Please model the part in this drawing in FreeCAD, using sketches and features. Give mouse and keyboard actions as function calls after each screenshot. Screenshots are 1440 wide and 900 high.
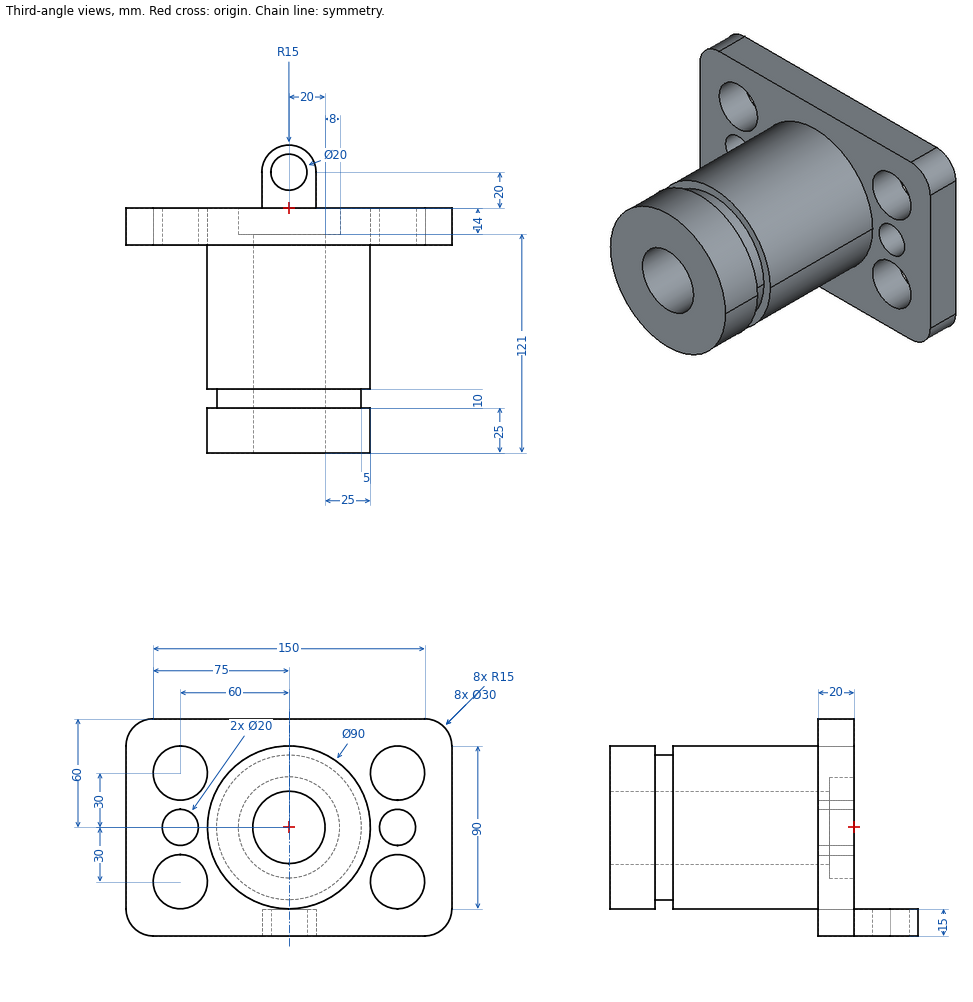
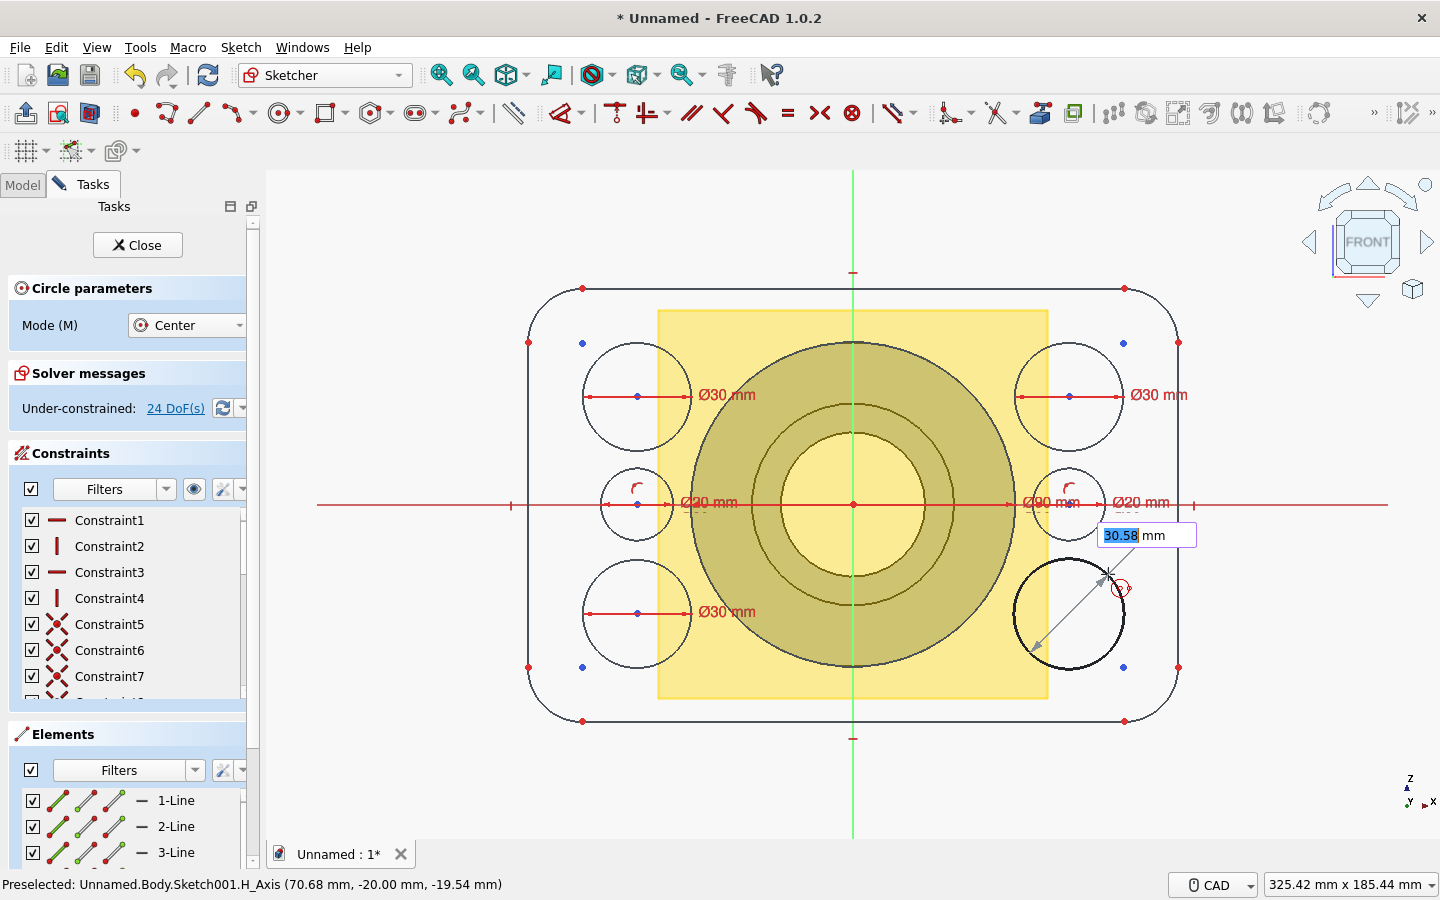
text(30)
key(Return)
key(Escape)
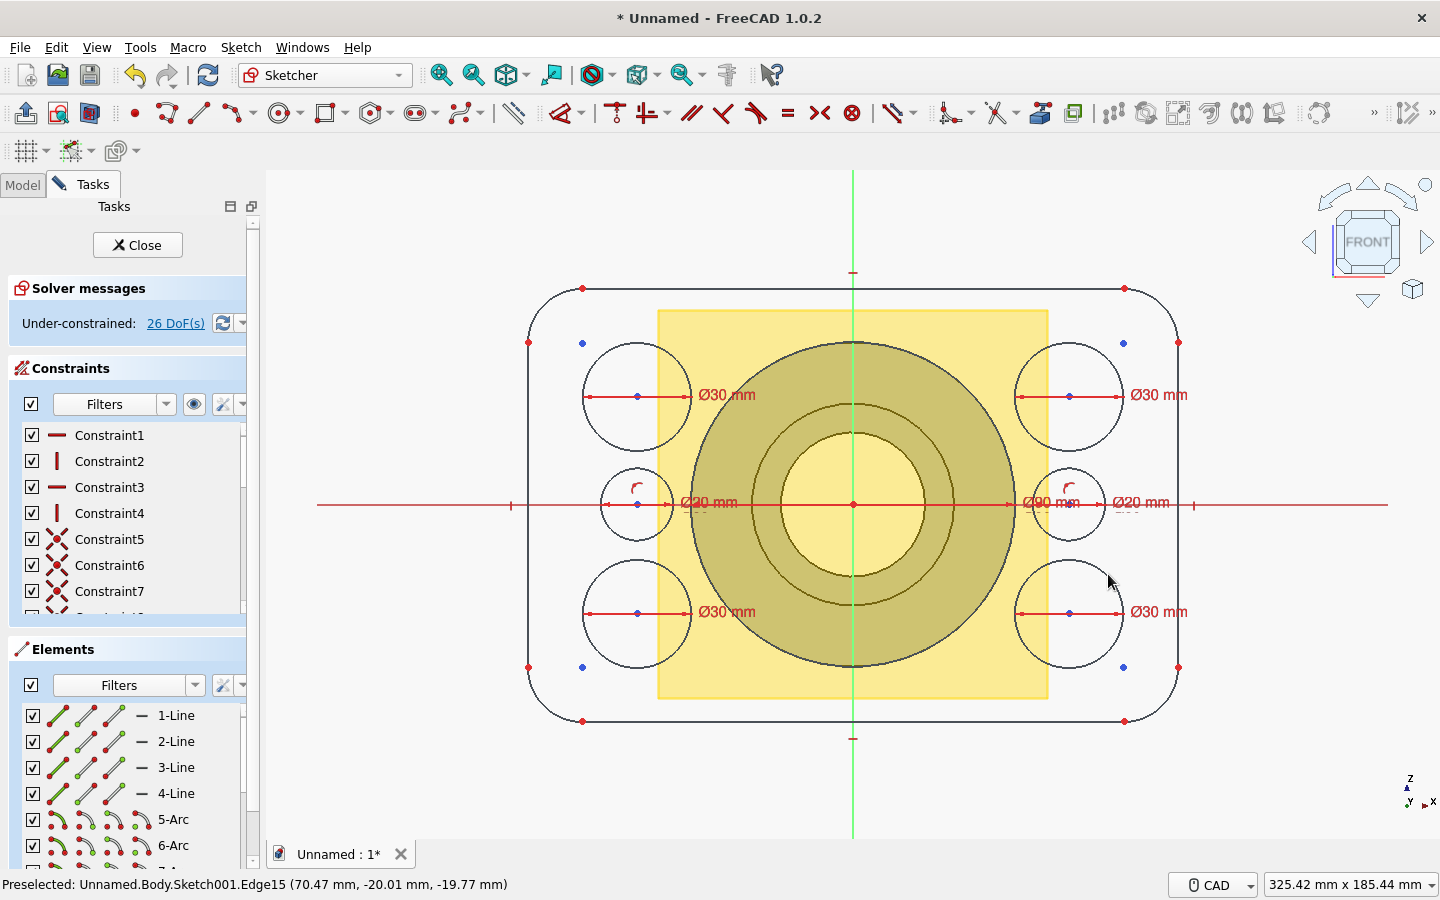
click(745, 289)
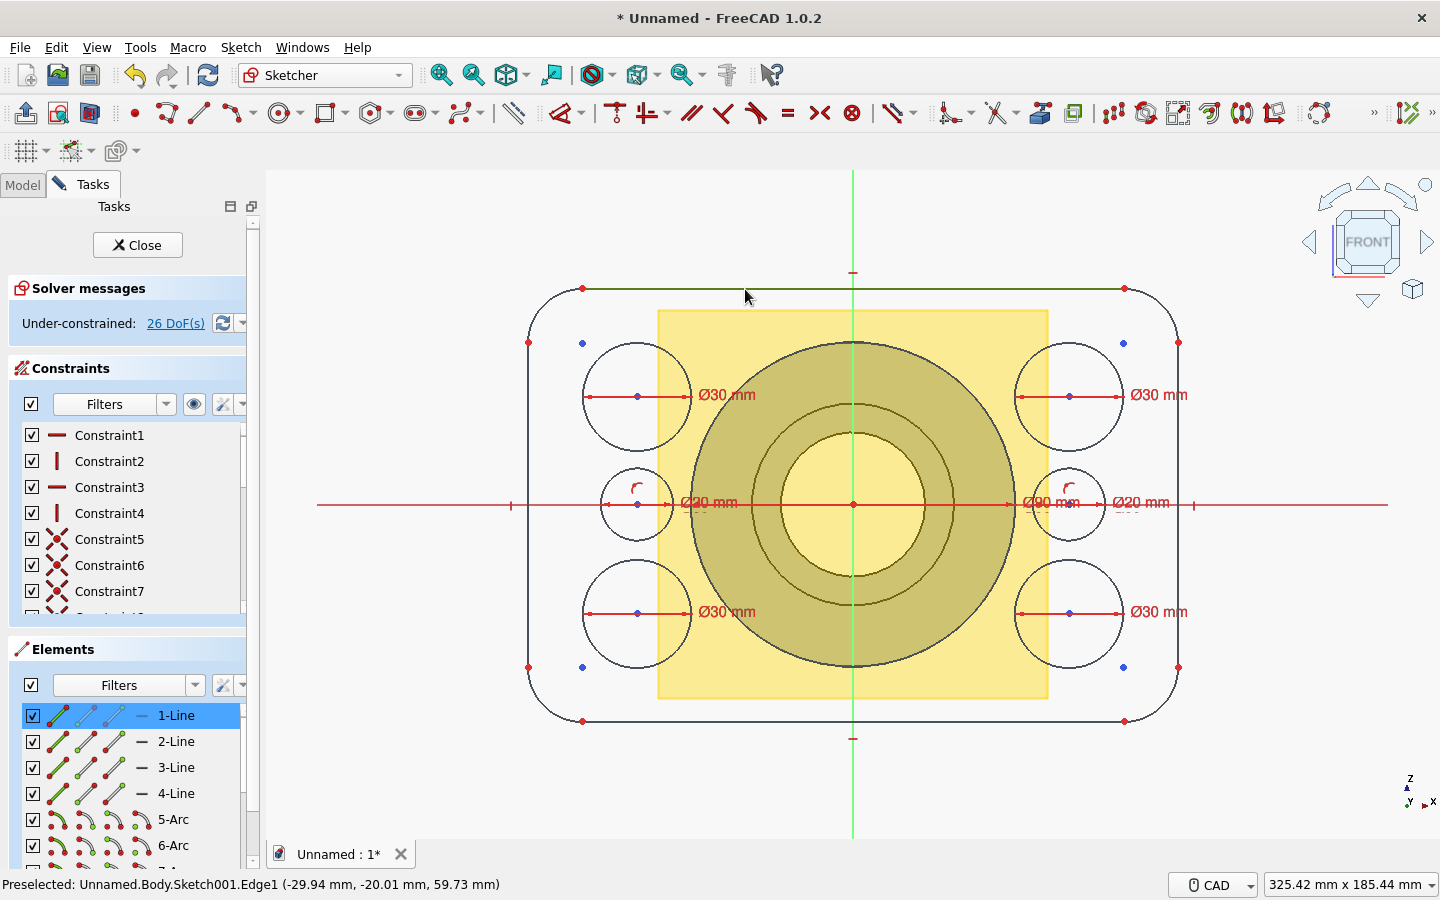
click(1172, 319)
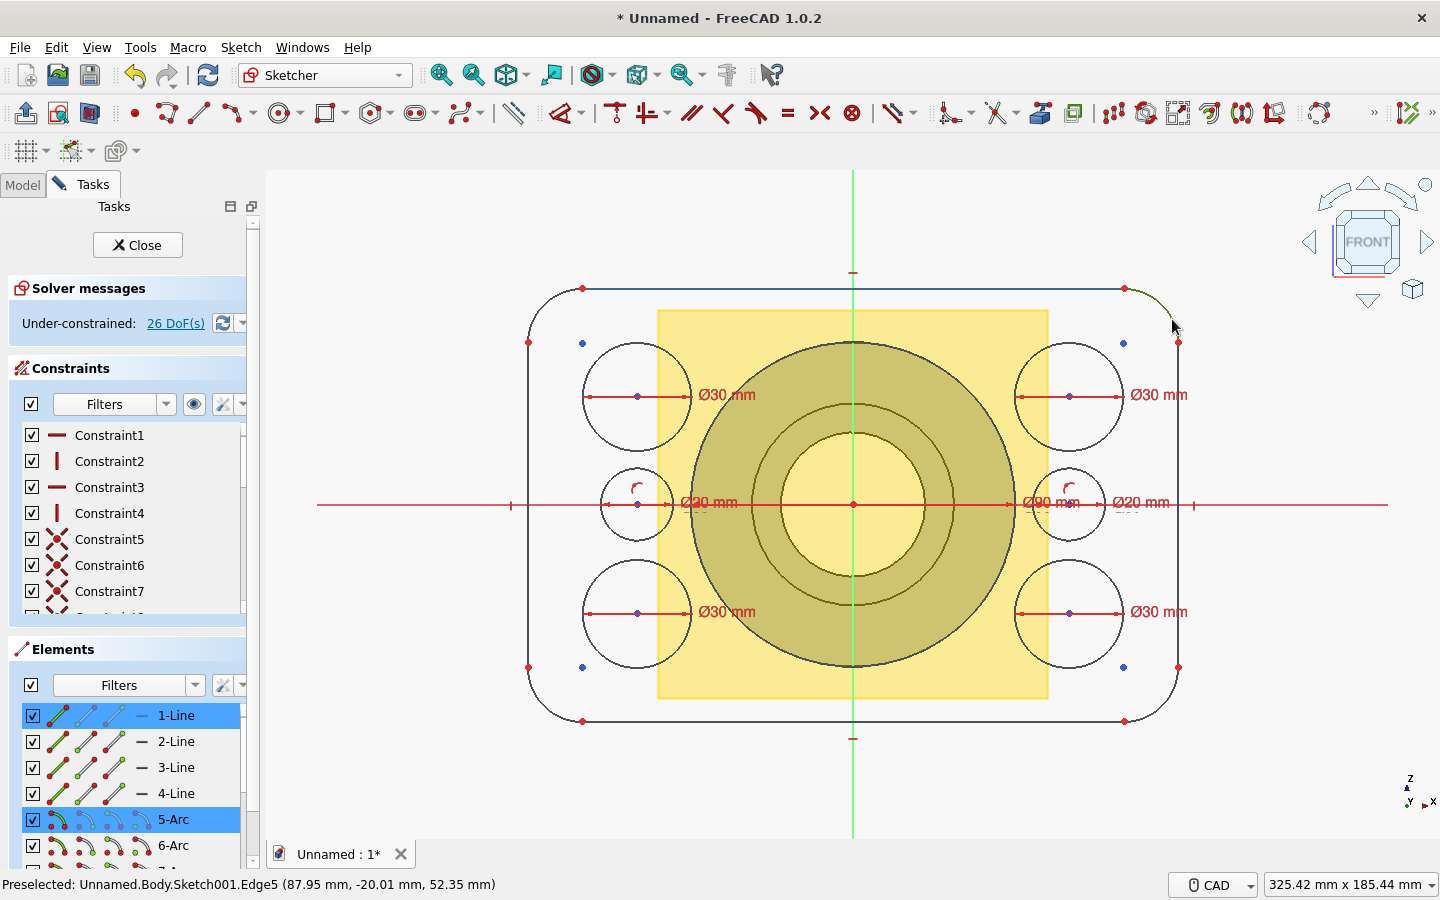
click(756, 114)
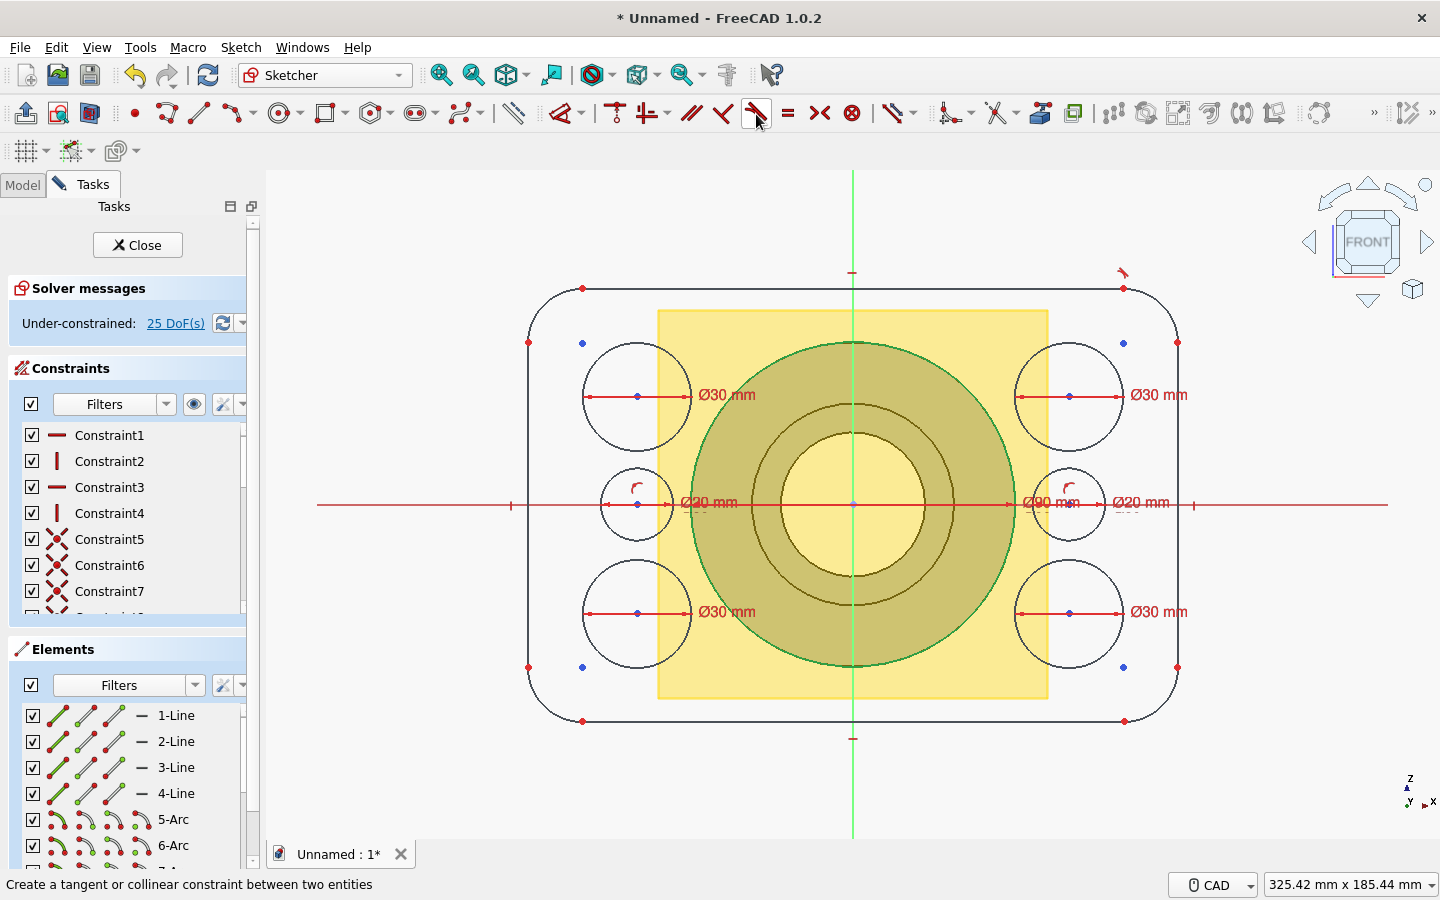
click(744, 289)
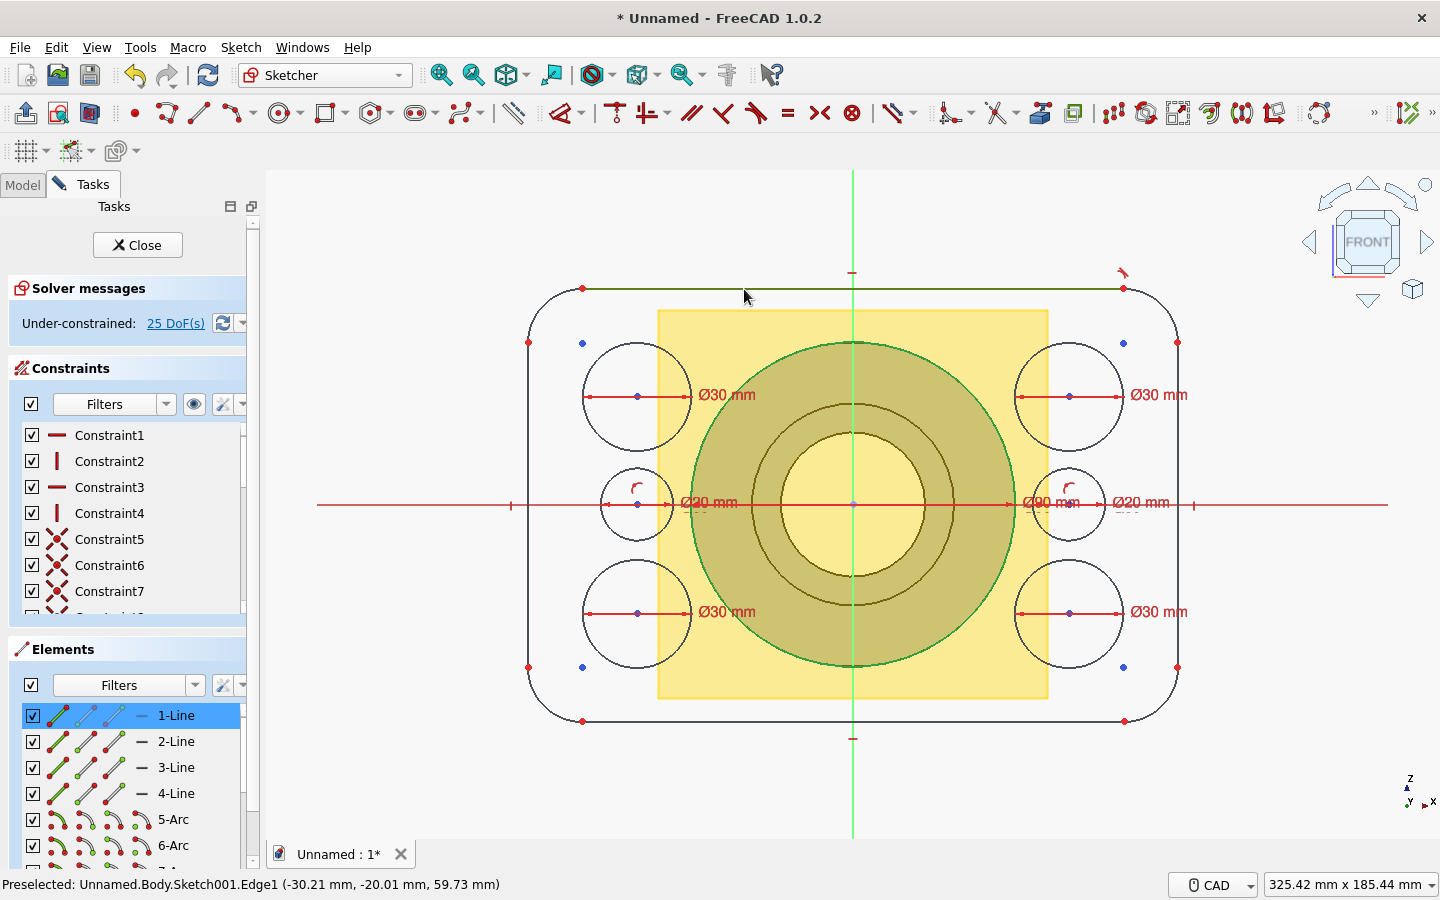
click(558, 295)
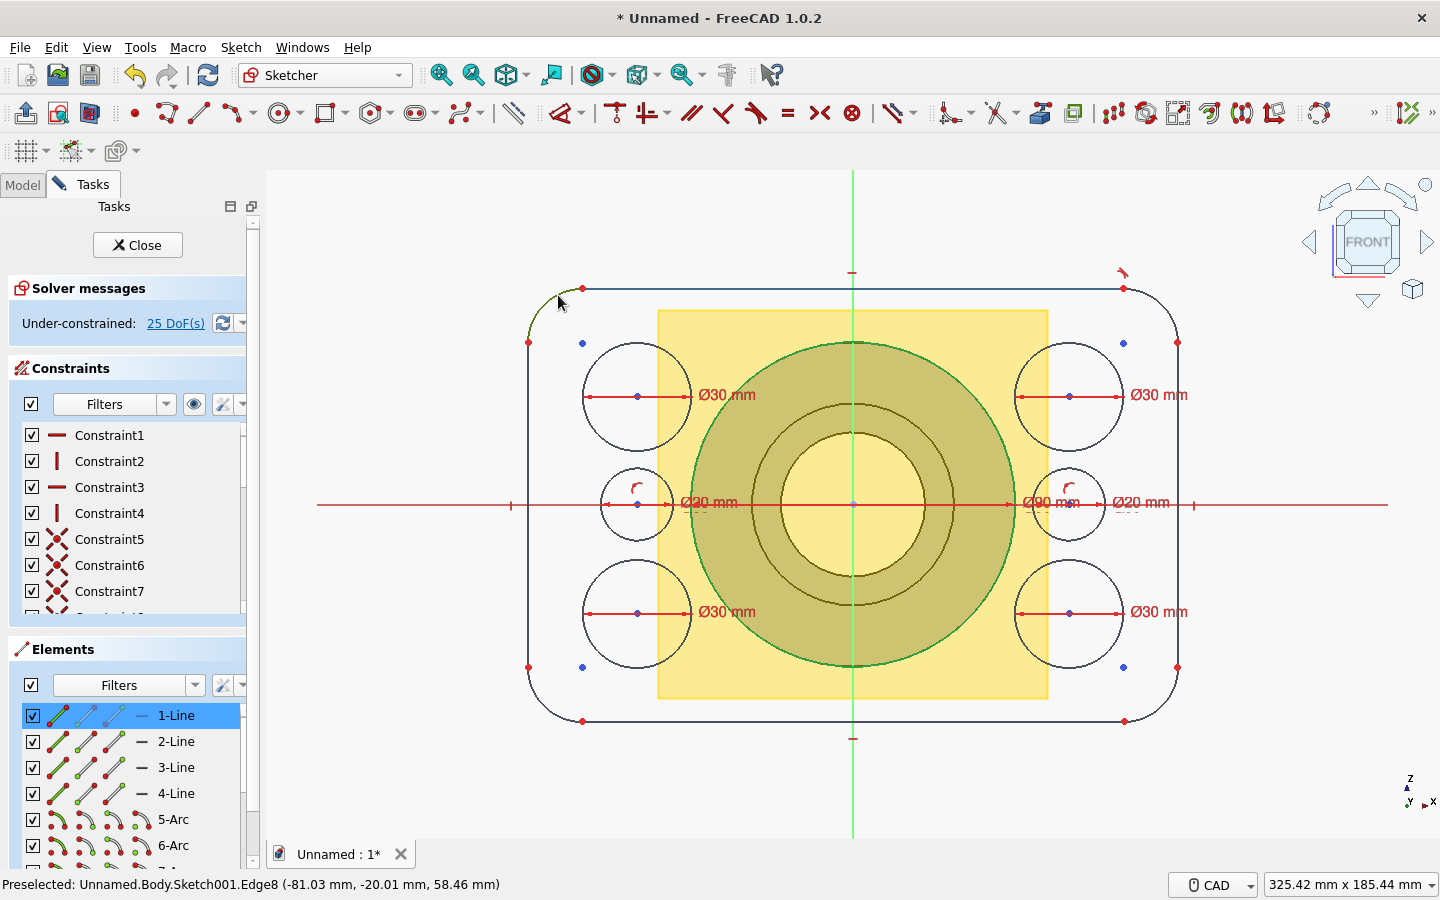
click(756, 114)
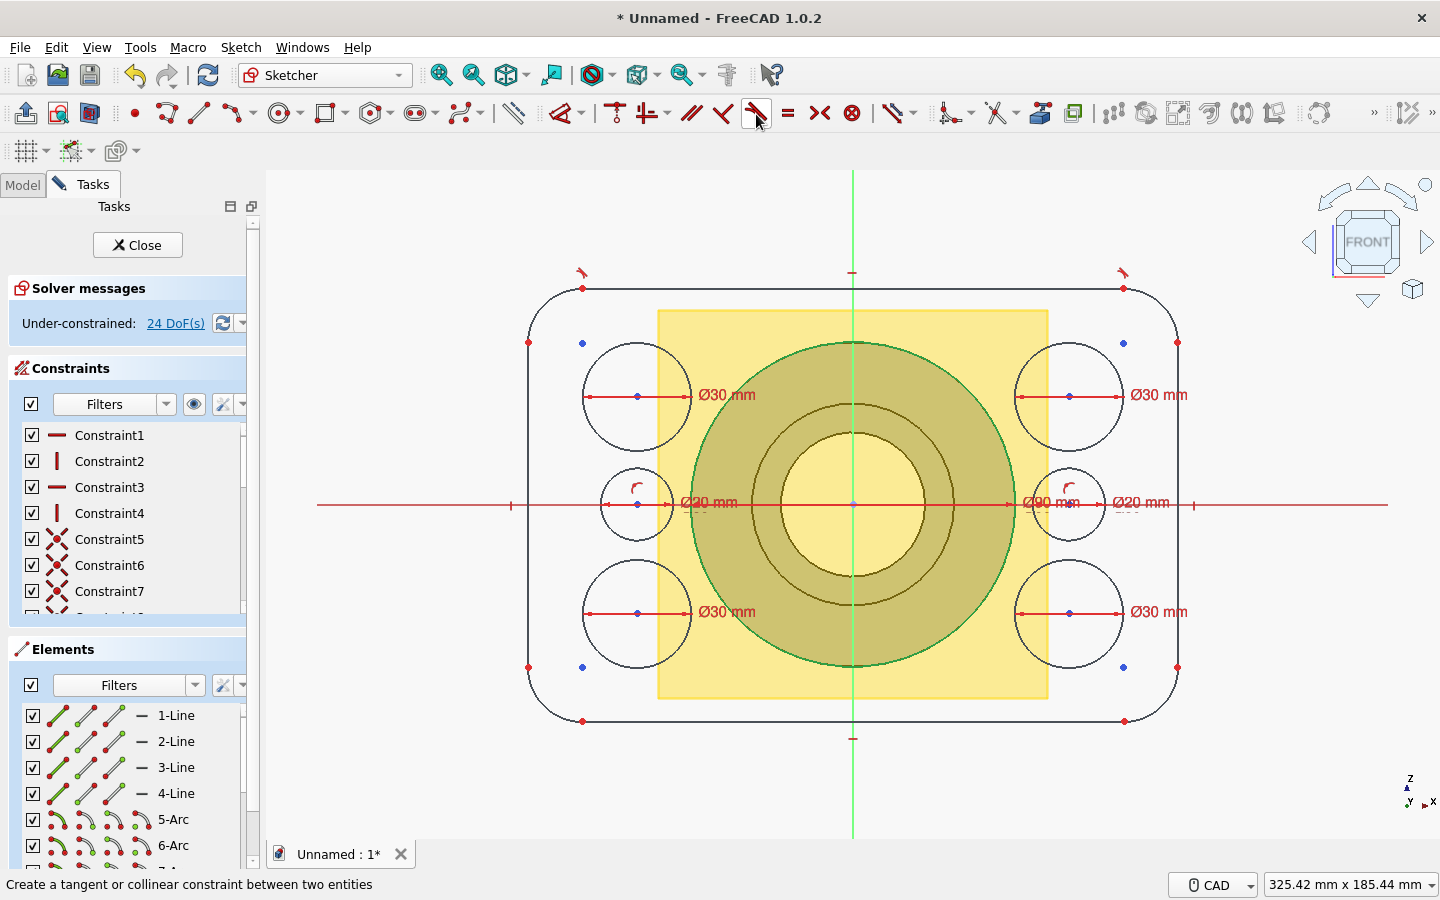
click(1178, 441)